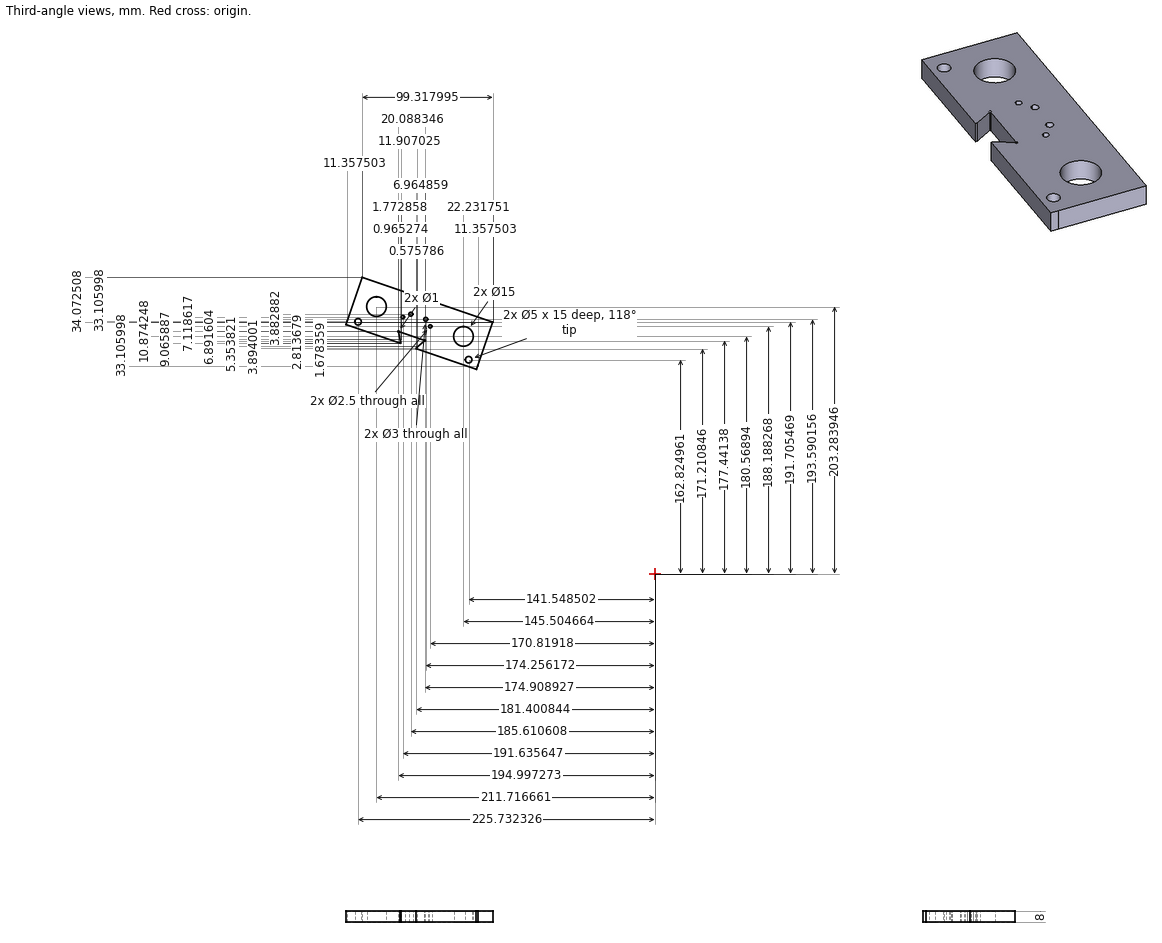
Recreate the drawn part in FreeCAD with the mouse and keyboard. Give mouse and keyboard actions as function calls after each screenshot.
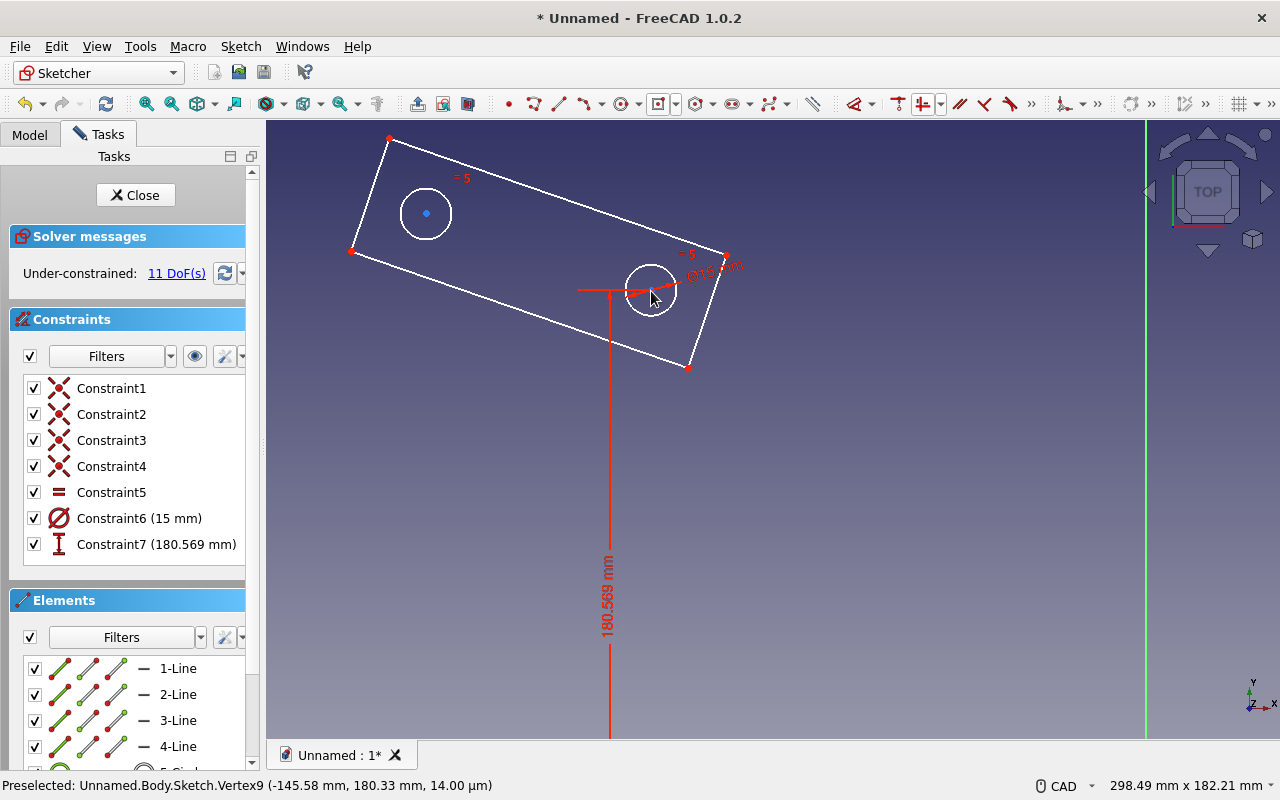
click(700, 334)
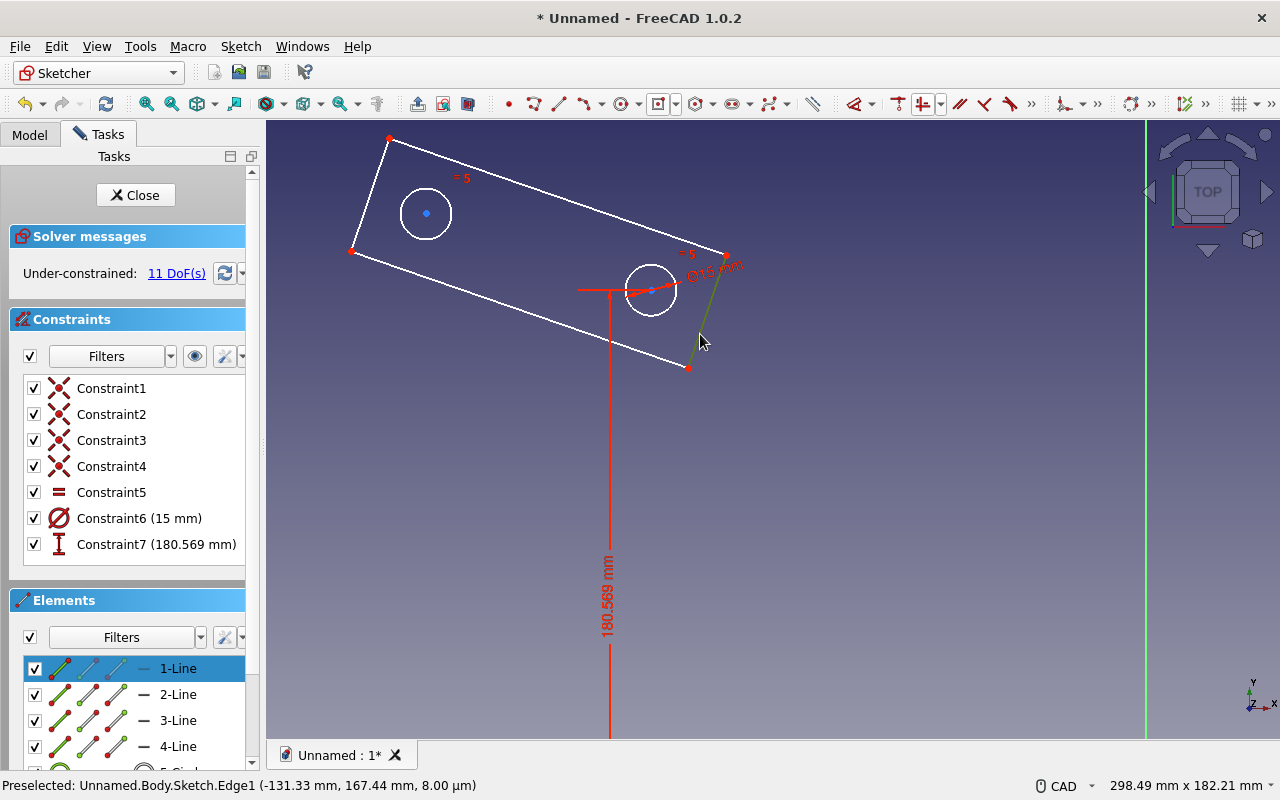
click(872, 104)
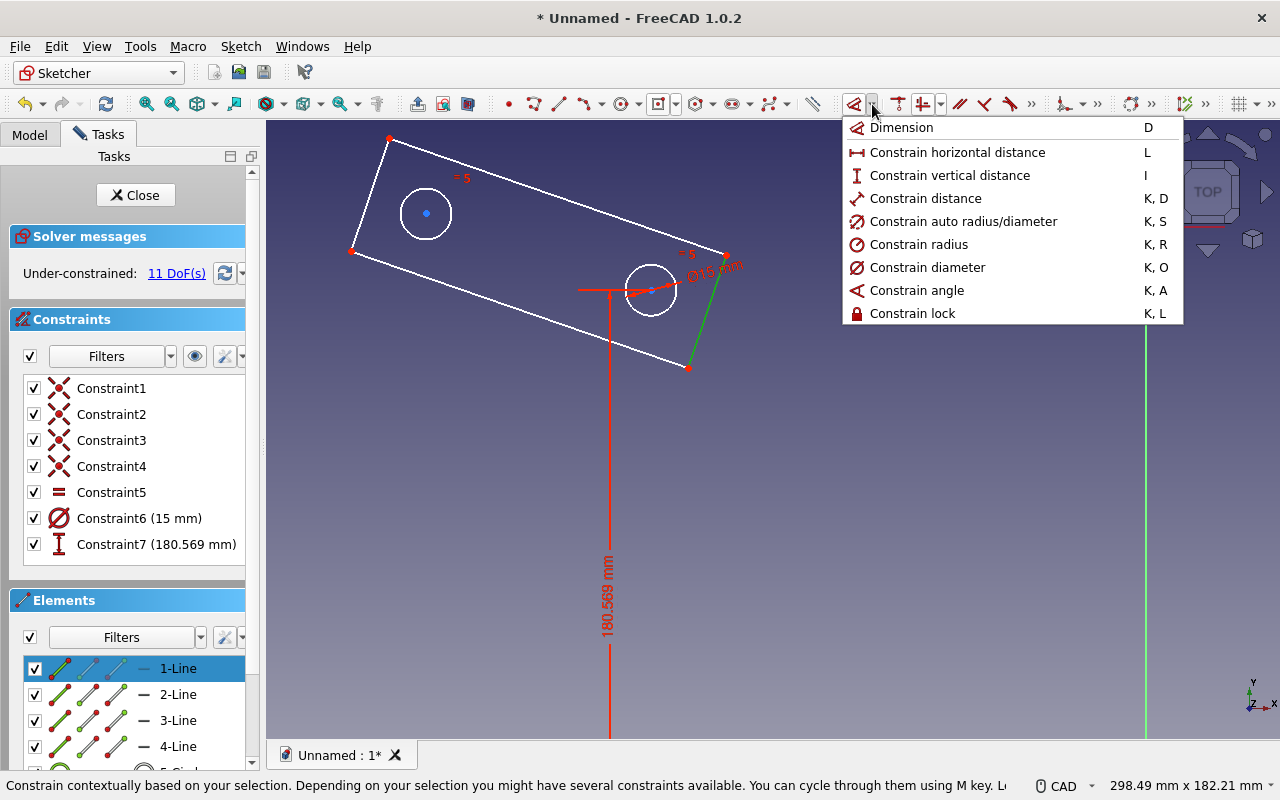
click(1013, 152)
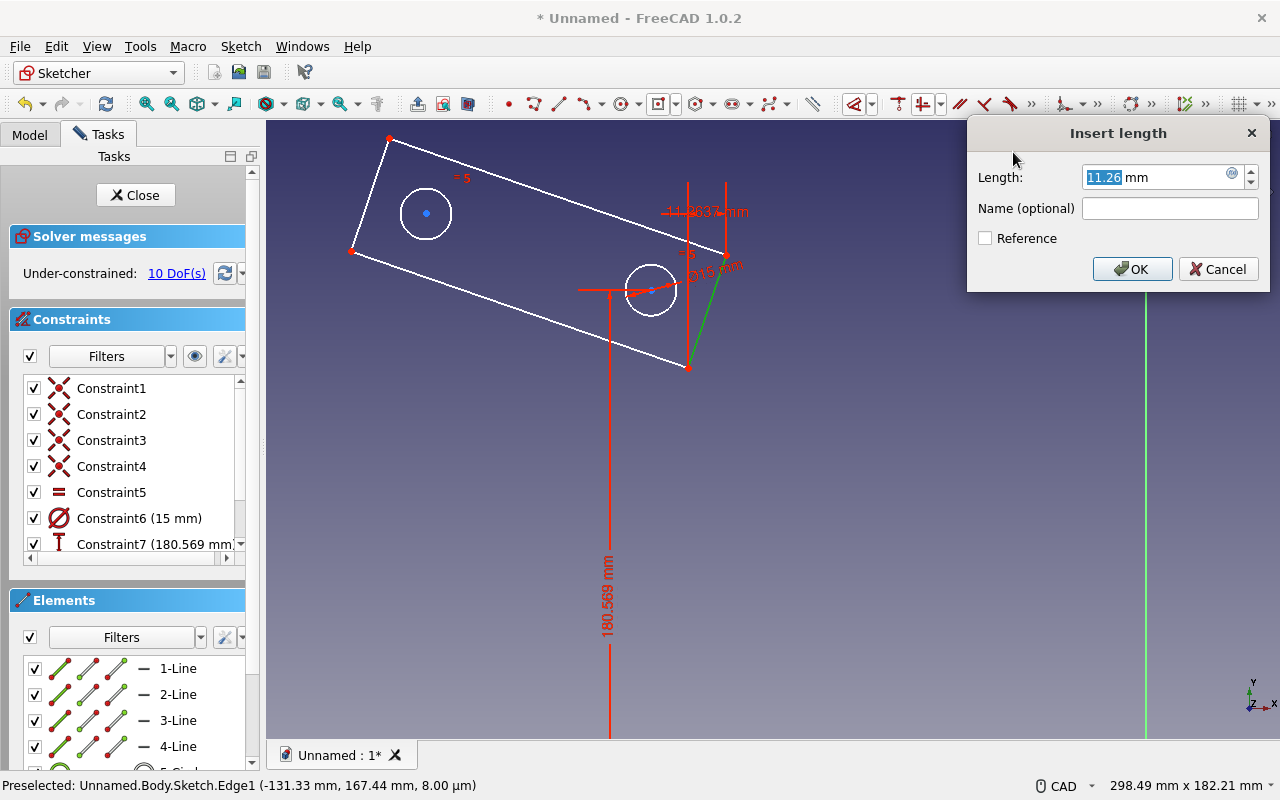
text(11.357503)
key(Return)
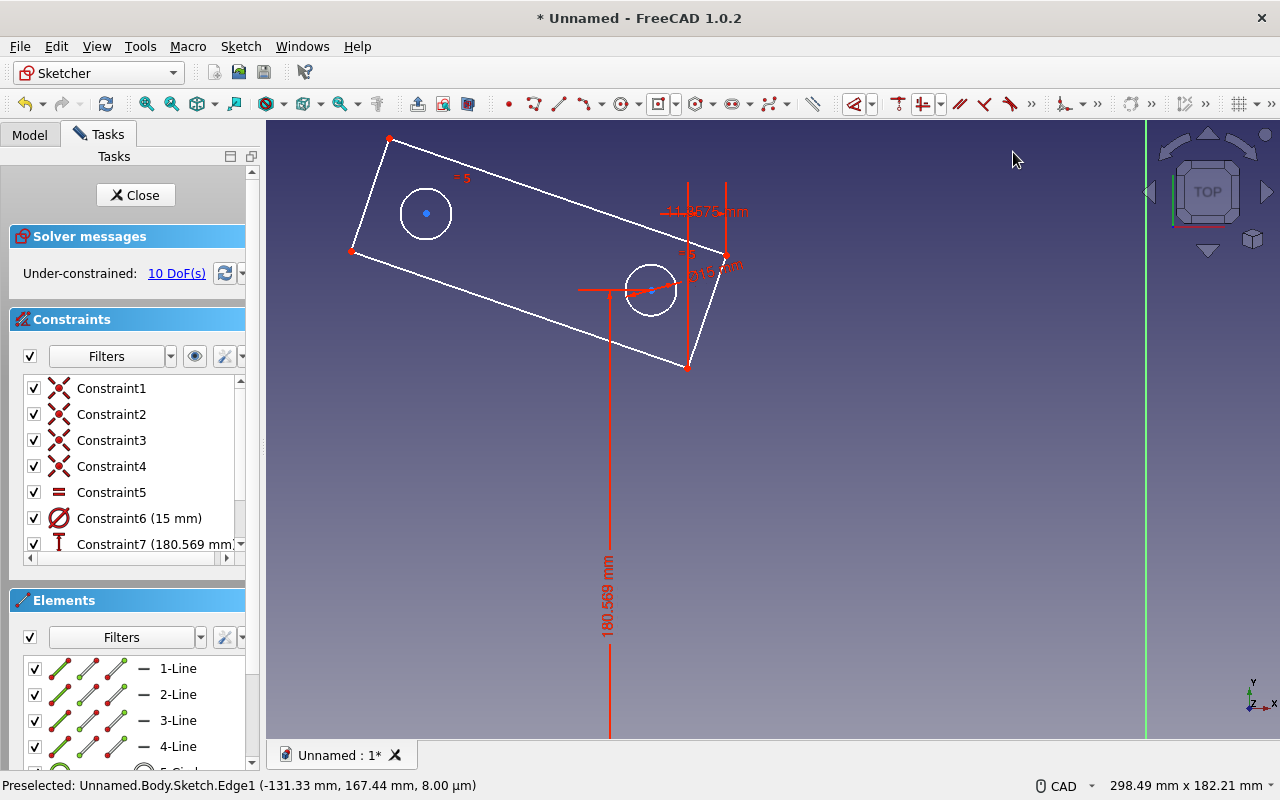
click(699, 334)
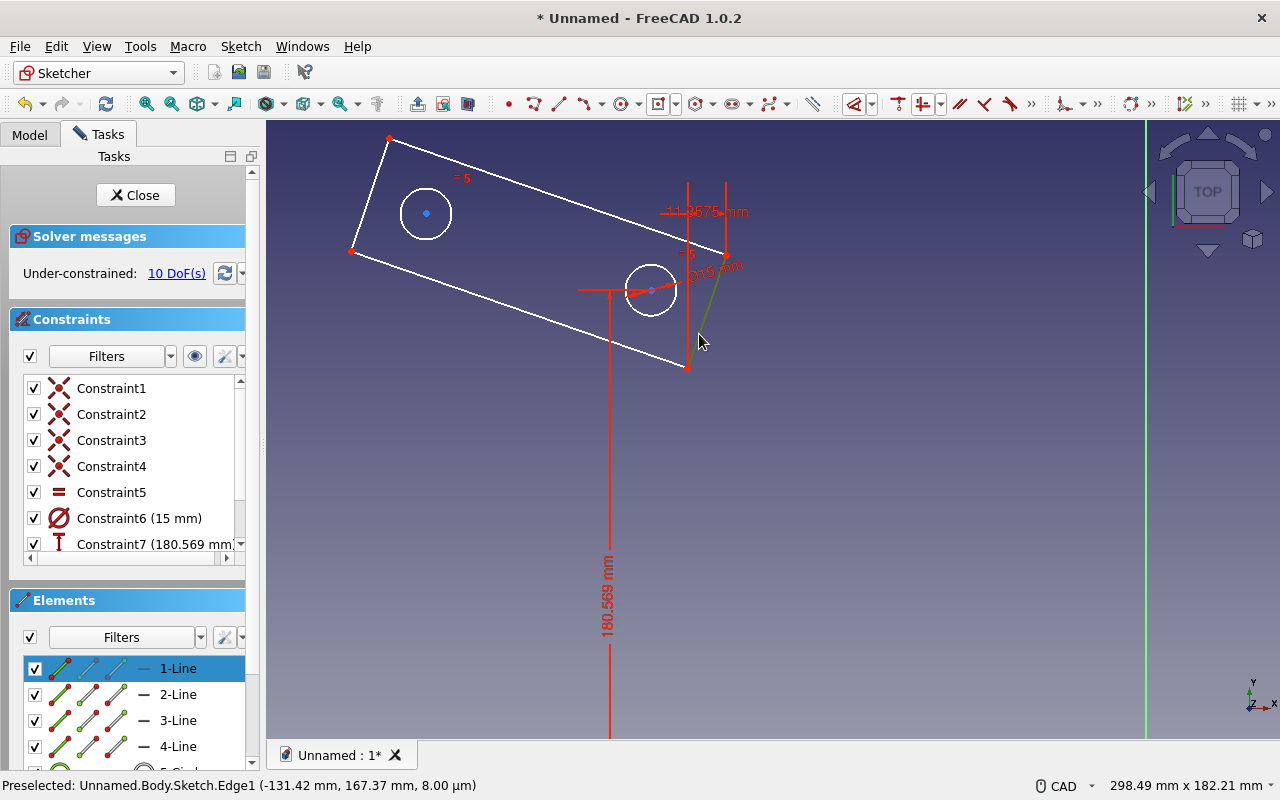
click(872, 104)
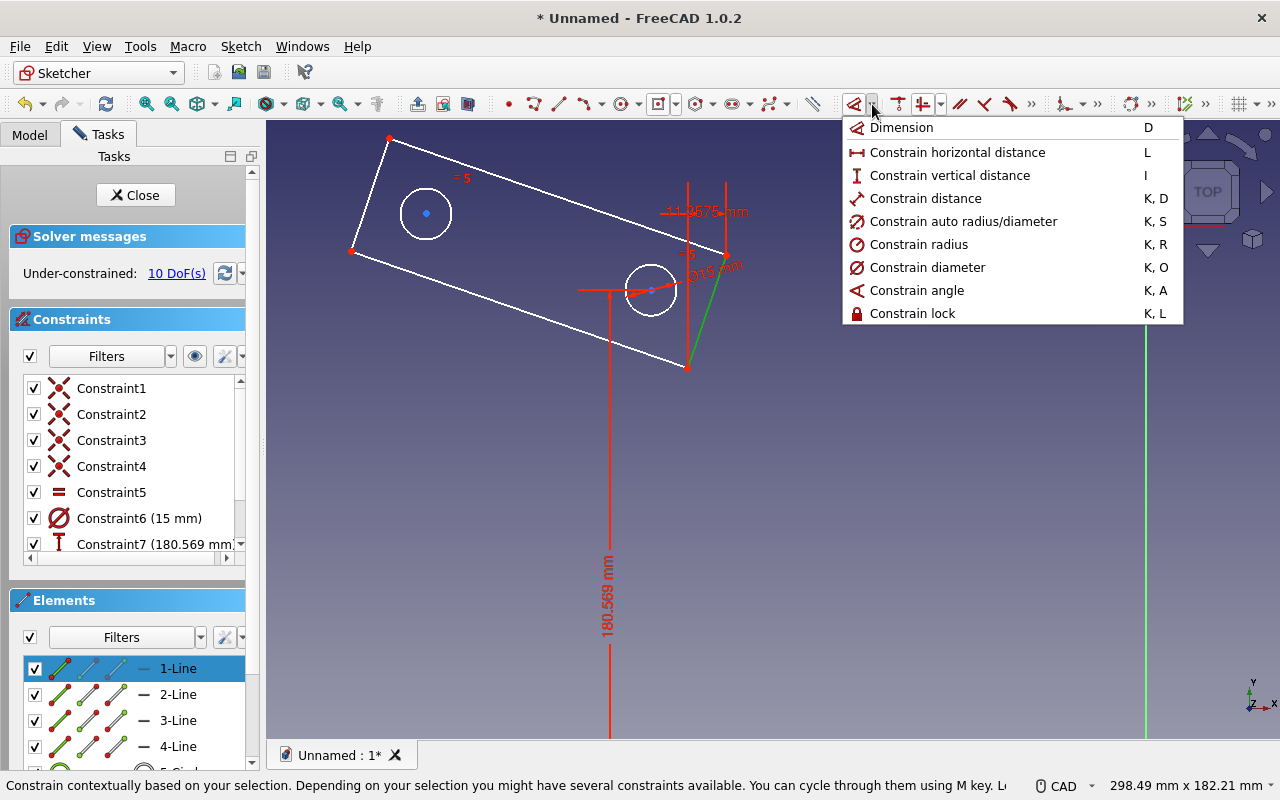
click(1013, 176)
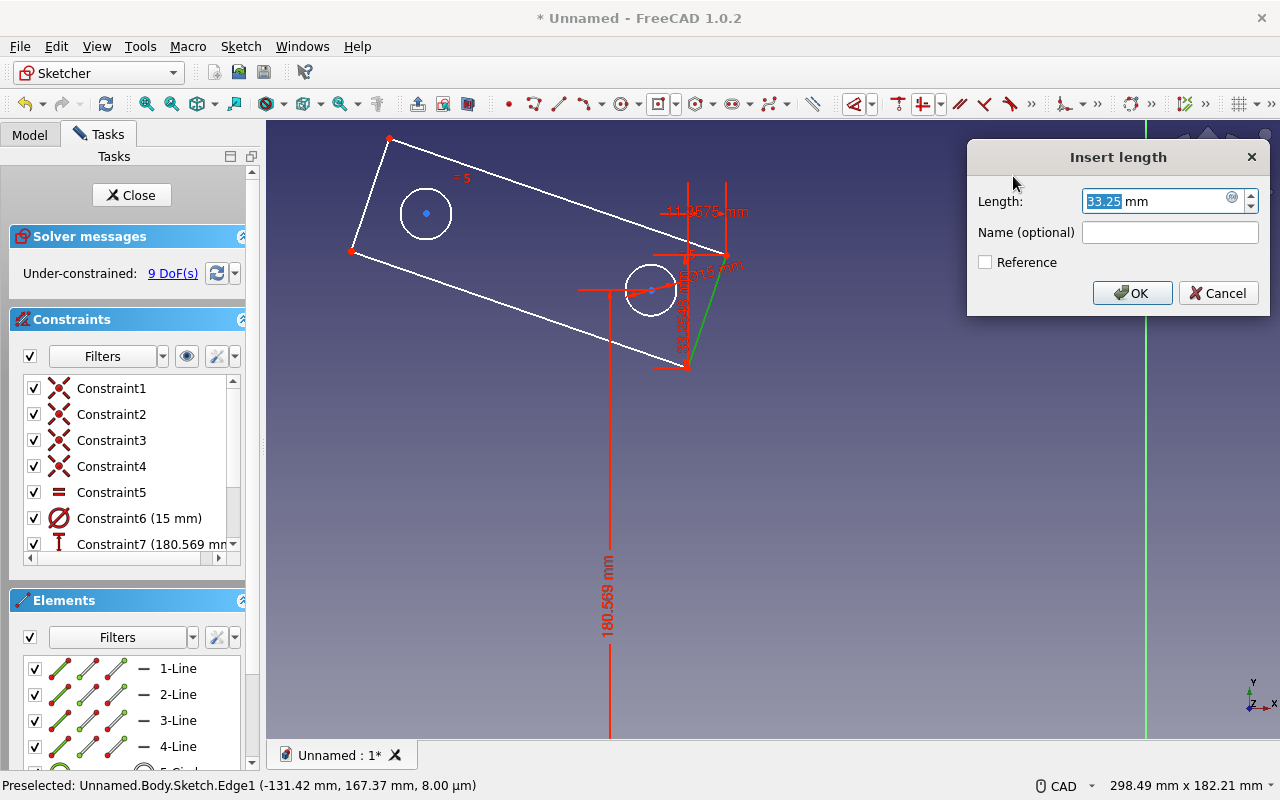
text(33.105998)
key(Return)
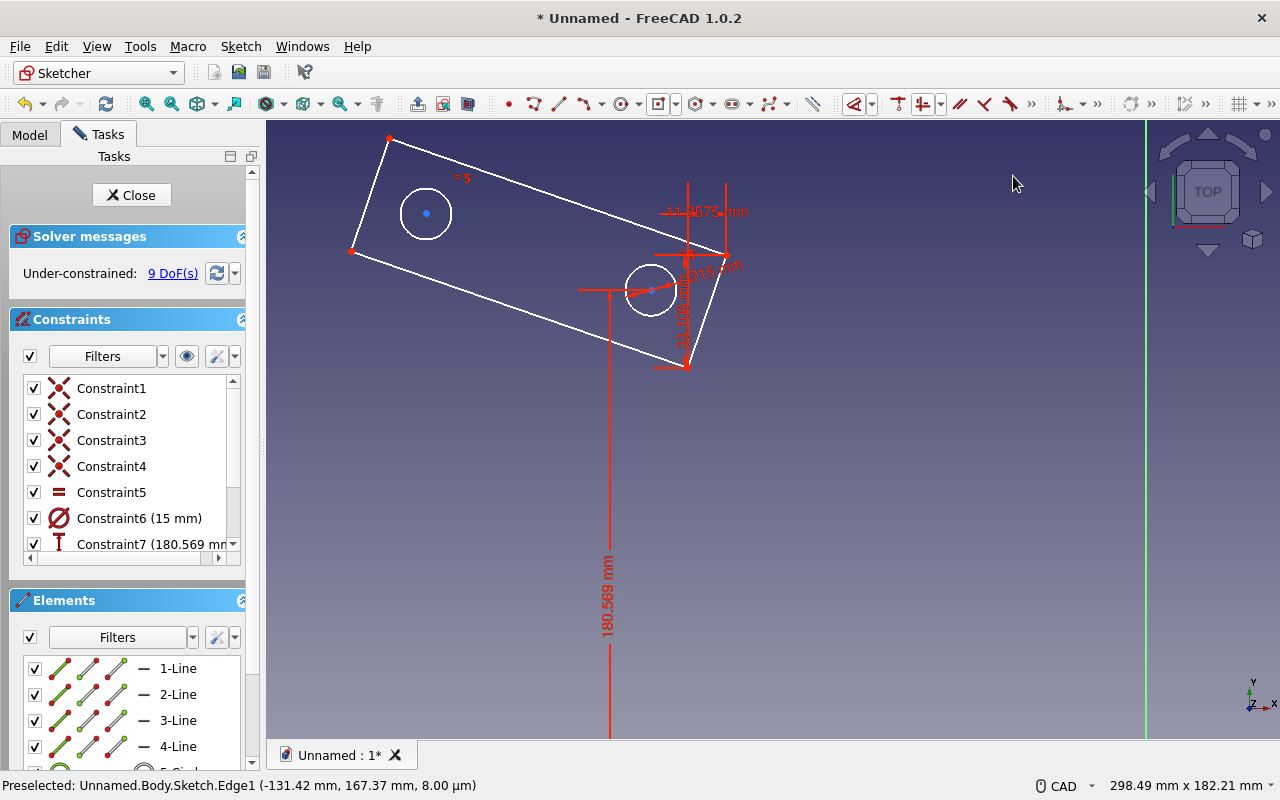
click(625, 220)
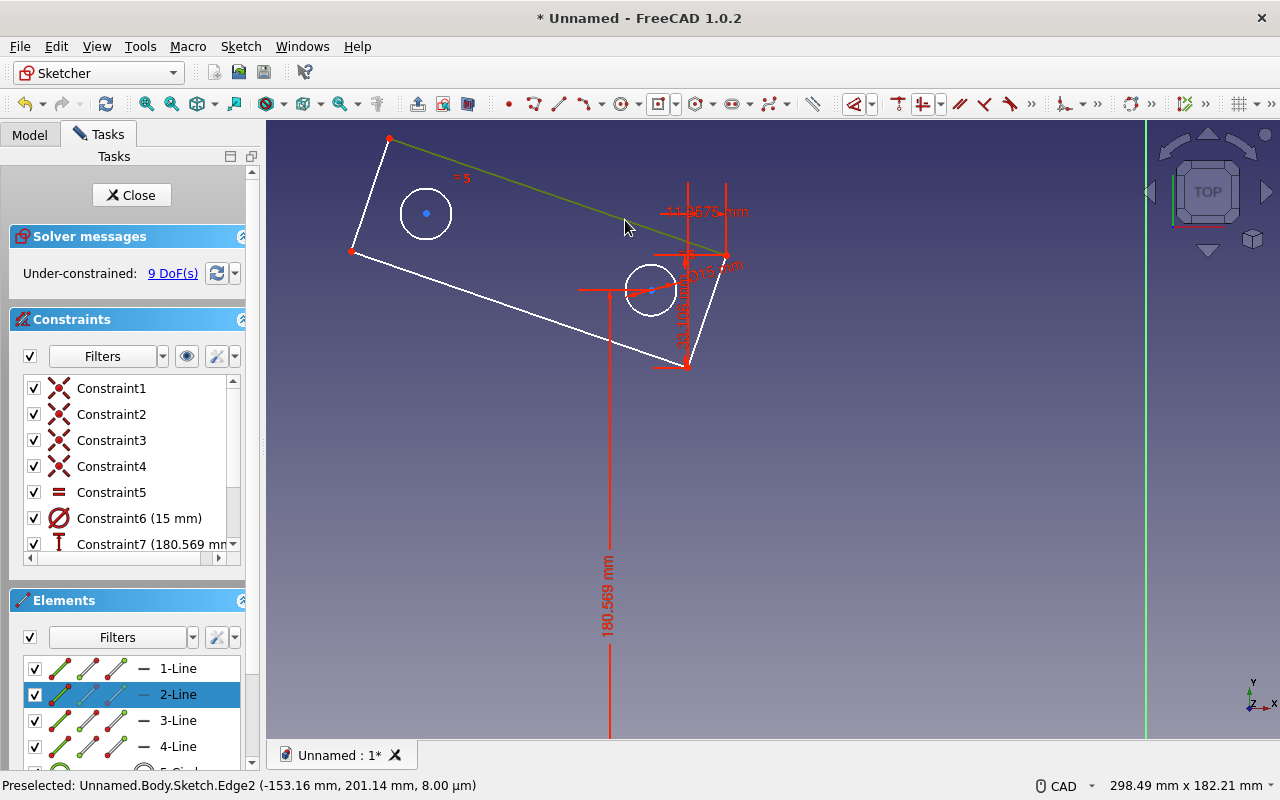
click(872, 104)